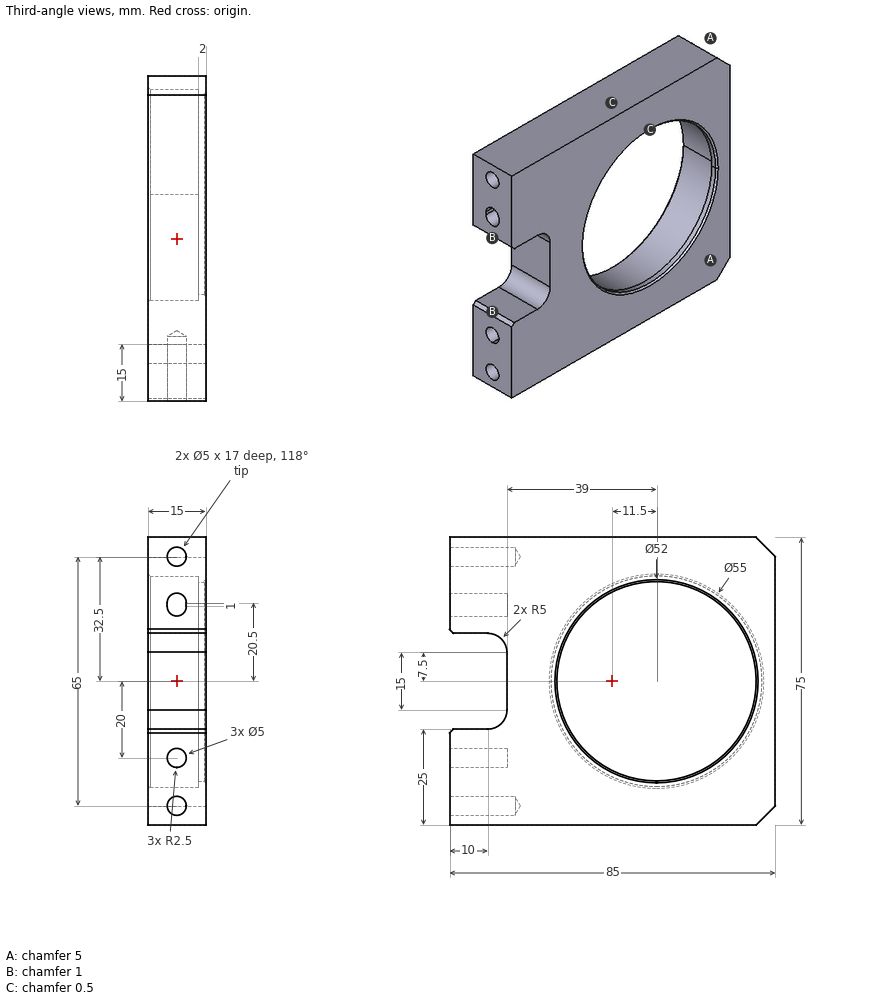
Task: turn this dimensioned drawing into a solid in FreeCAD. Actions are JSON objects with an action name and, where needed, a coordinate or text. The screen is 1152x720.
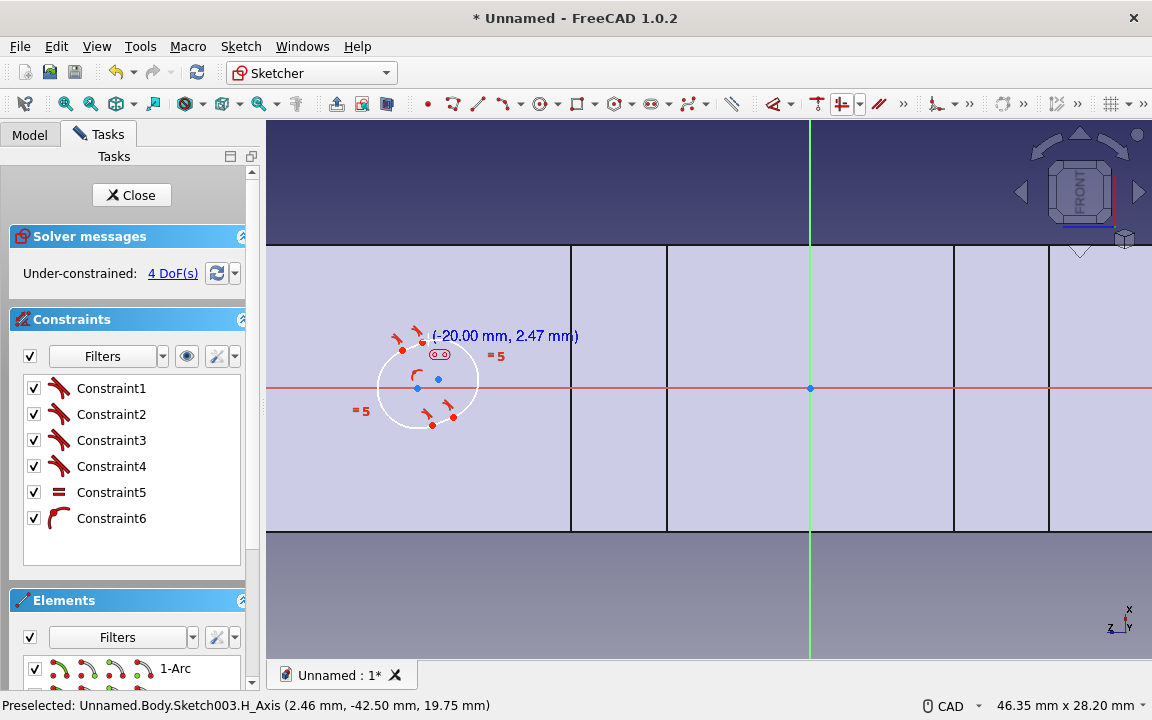
{"action": "left_click", "coordinate": [540, 104]}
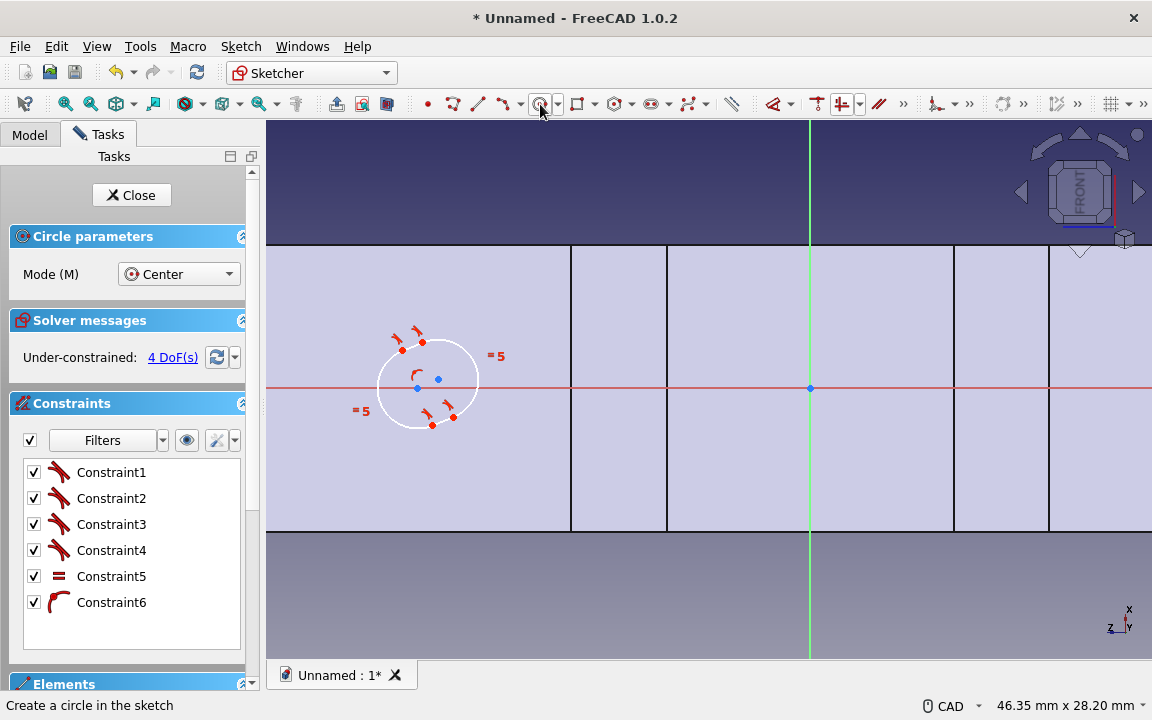
{"action": "scroll", "coordinate": [440, 391], "scroll_direction": "down", "scroll_amount": 3}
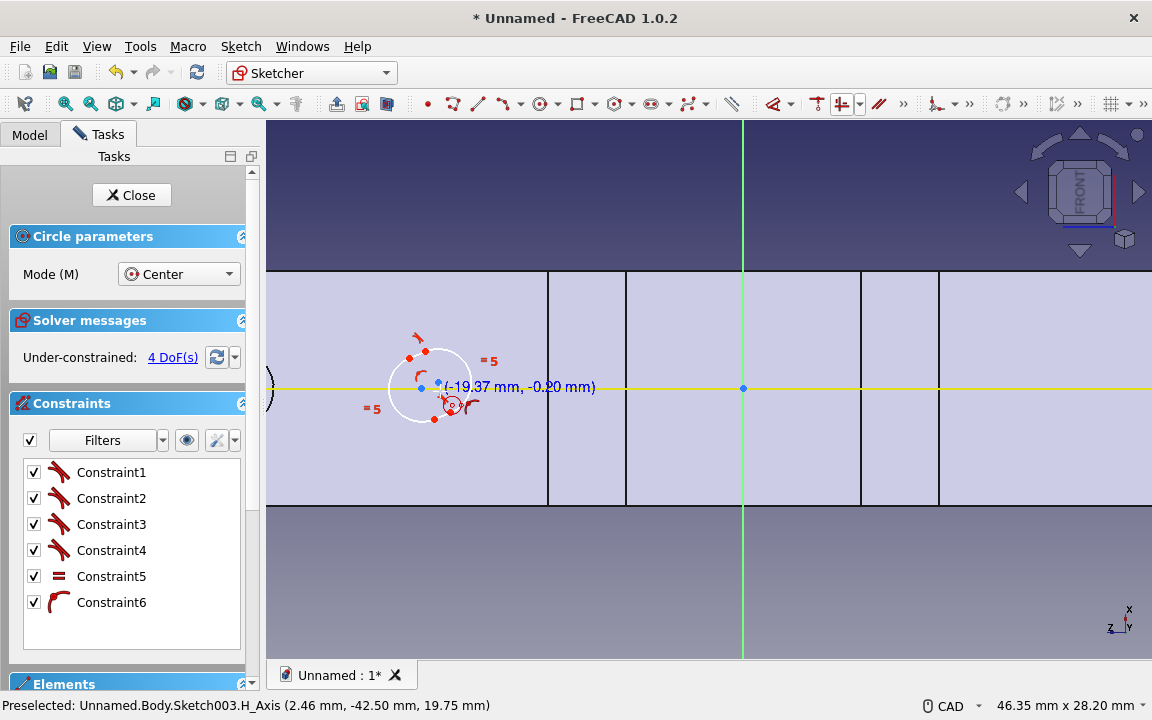
{"action": "left_click", "coordinate": [853, 390]}
{"action": "mouse_move", "coordinate": [872, 371]}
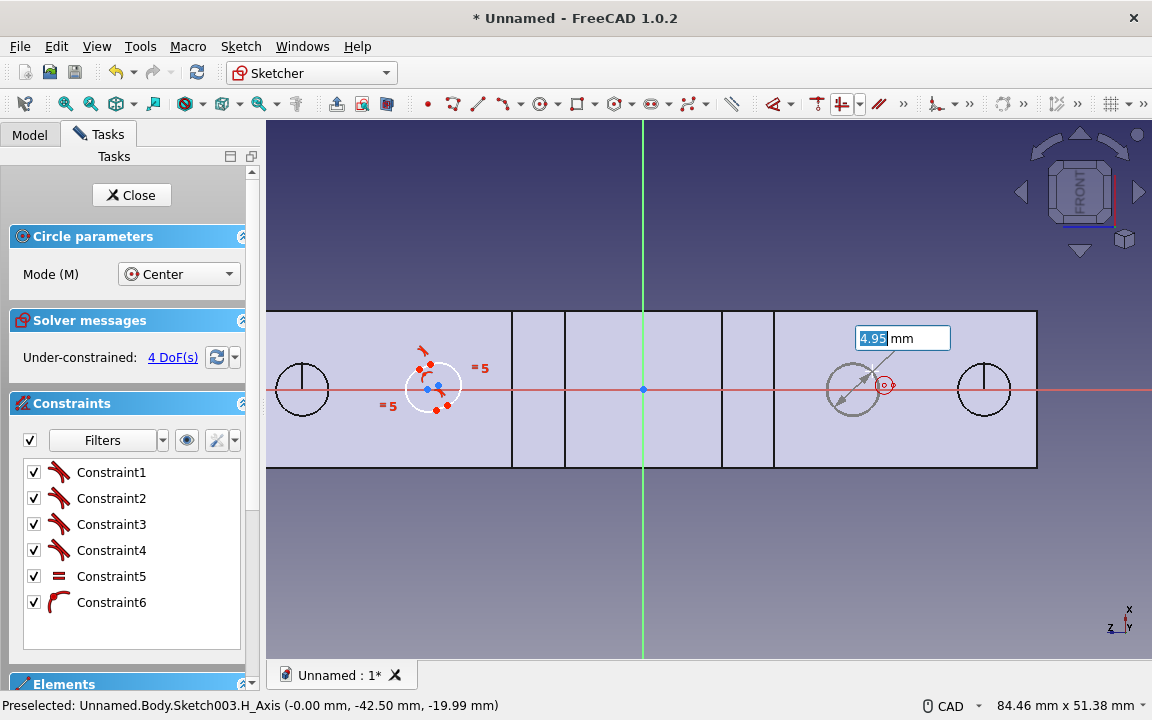
{"action": "type", "text": "5"}
{"action": "key", "text": "Return"}
{"action": "key", "text": "Escape"}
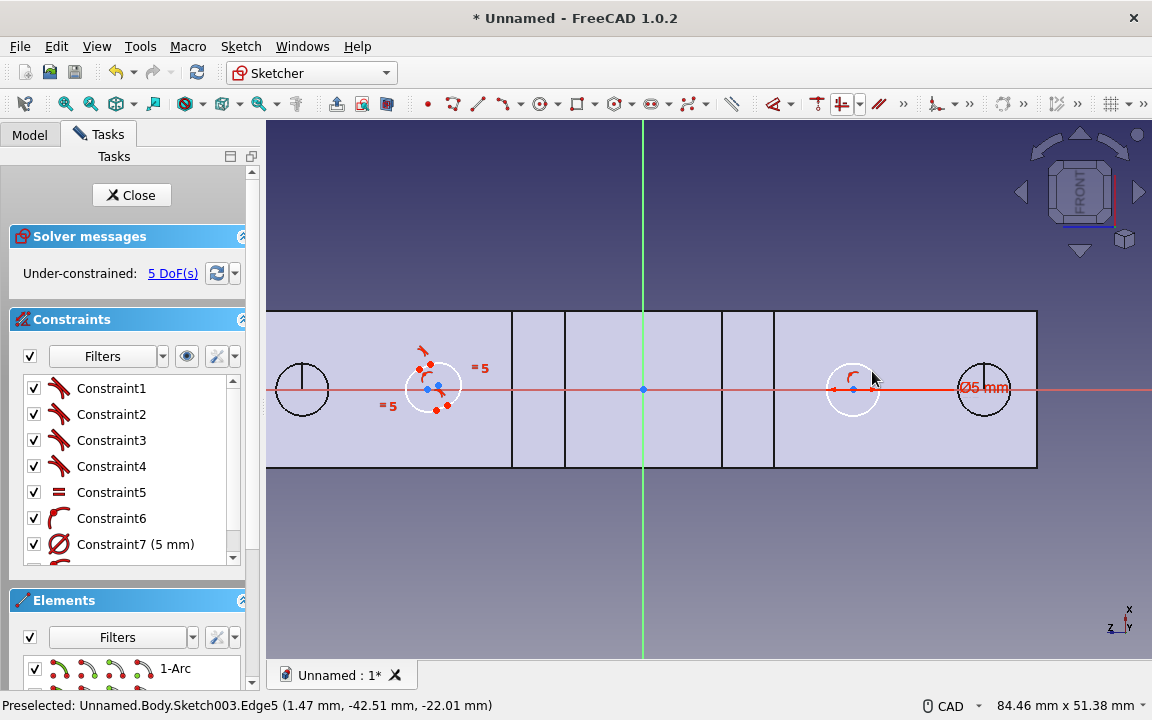
{"action": "left_click", "coordinate": [439, 385]}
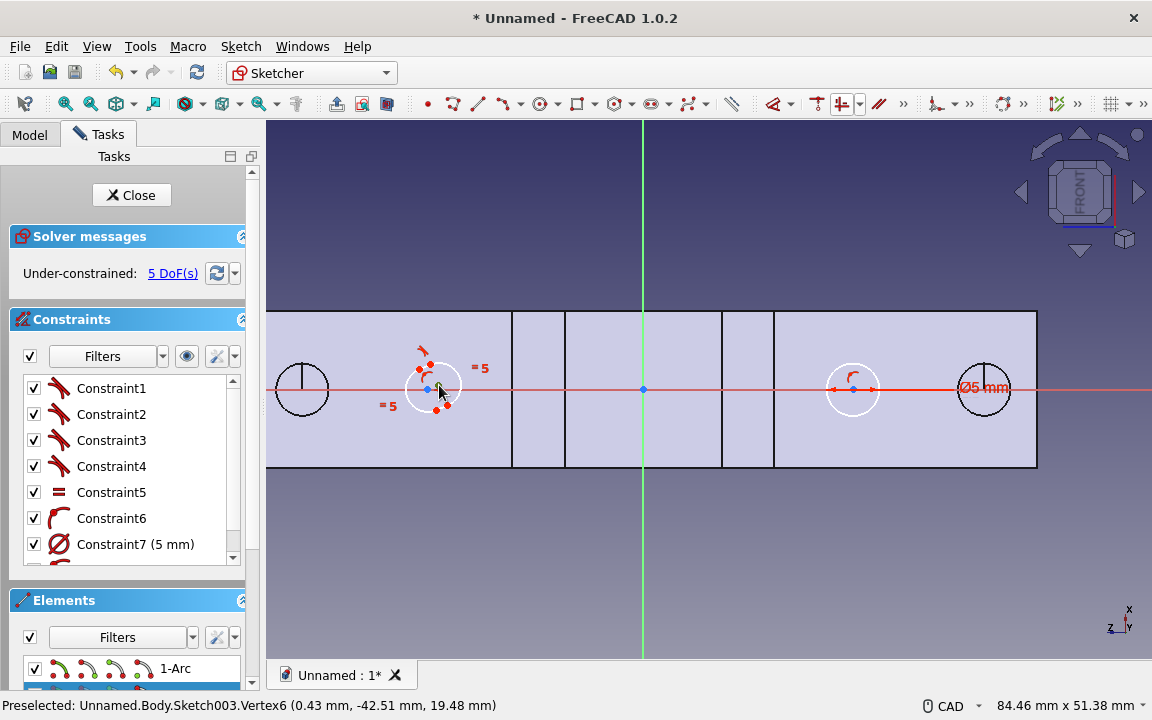
{"action": "left_click", "coordinate": [344, 390]}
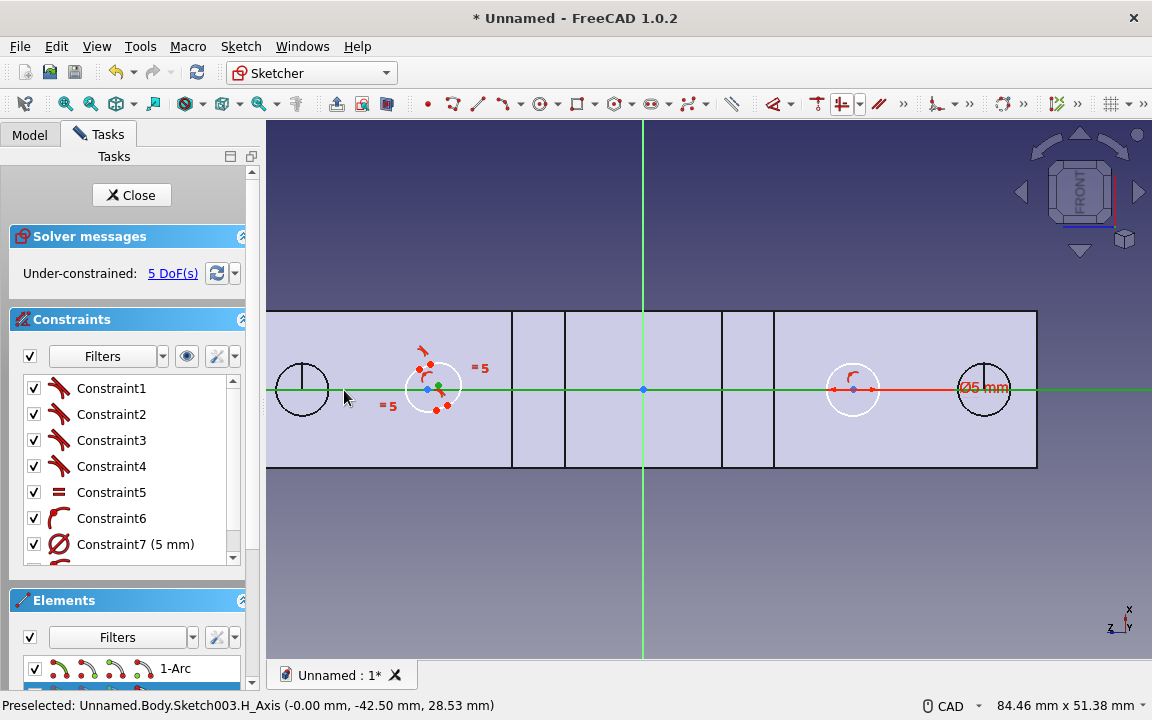
{"action": "left_click", "coordinate": [817, 104]}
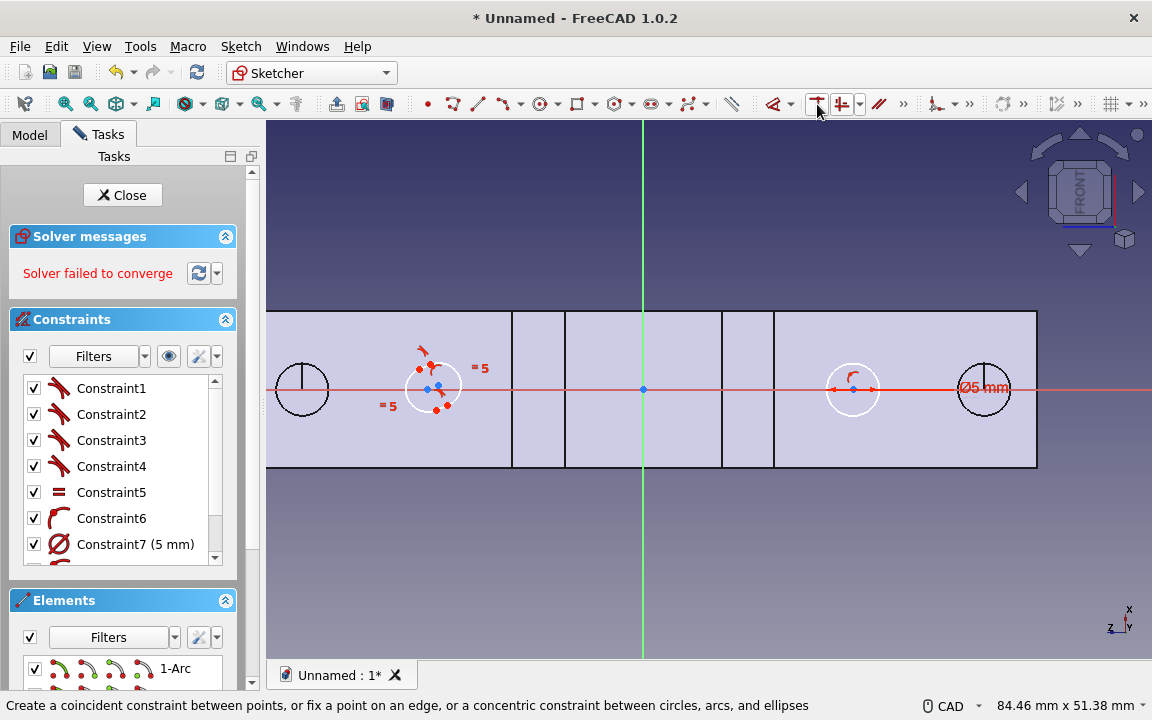
{"action": "left_click", "coordinate": [772, 104]}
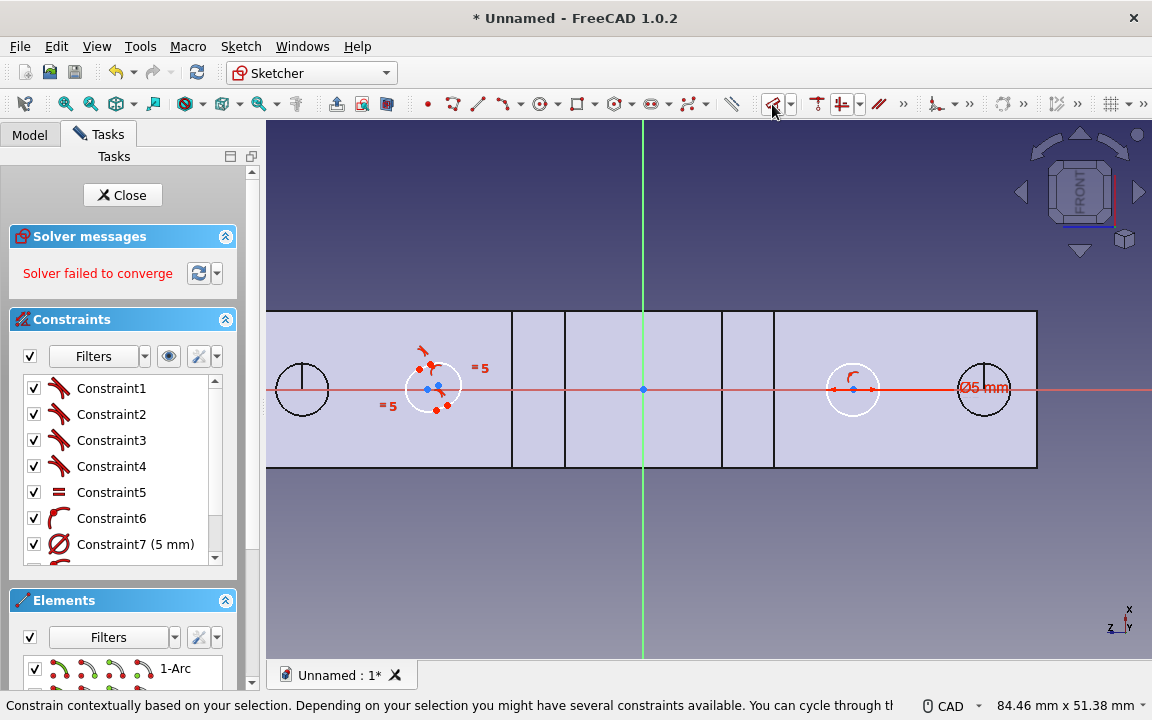
{"action": "scroll", "coordinate": [416, 408], "scroll_direction": "up", "scroll_amount": 3}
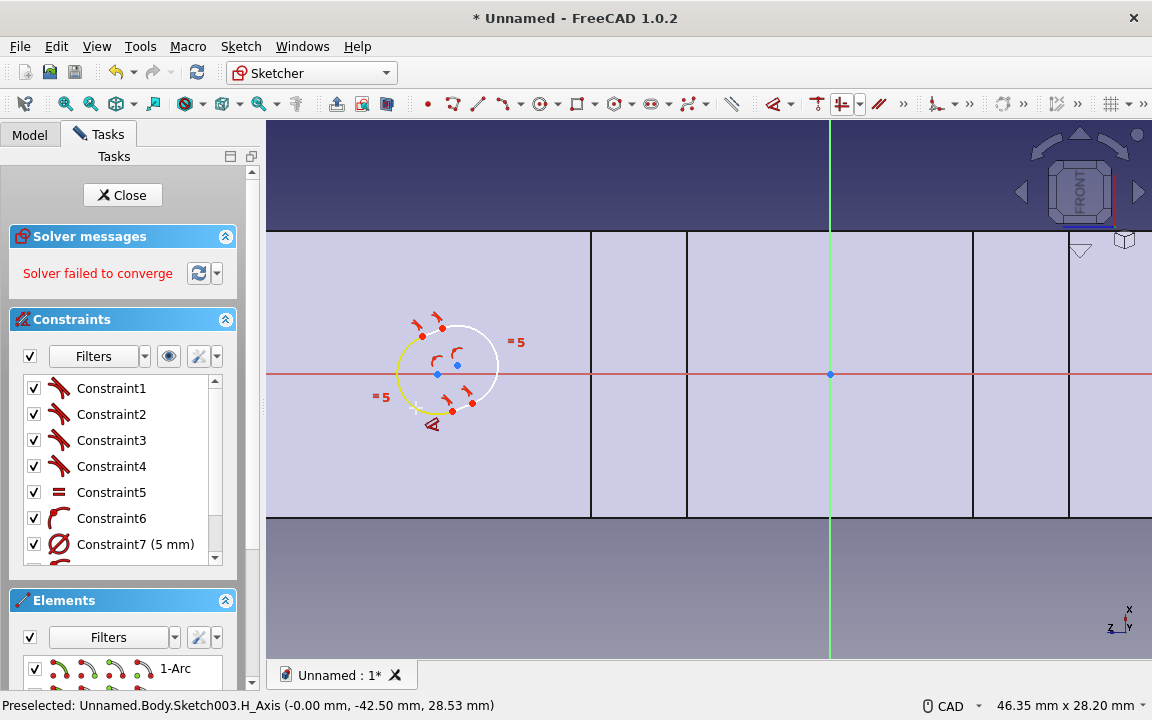
{"action": "left_click", "coordinate": [416, 408]}
{"action": "left_click", "coordinate": [399, 435]}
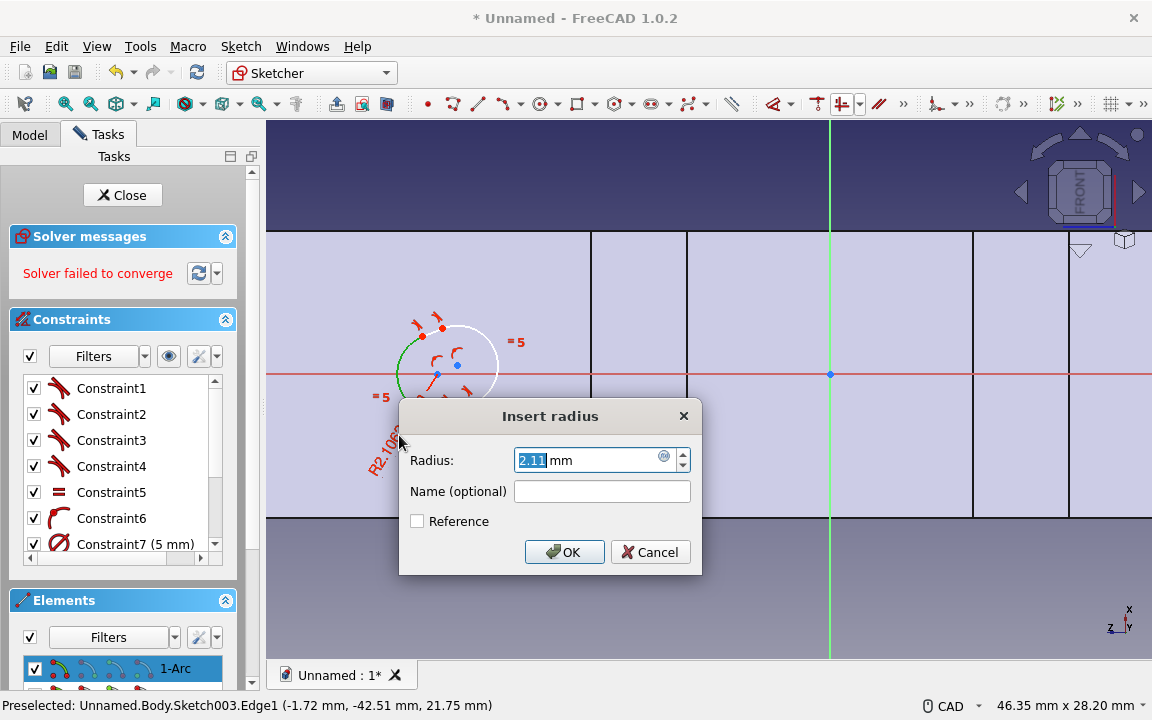
{"action": "type", "text": "2.5"}
{"action": "key", "text": "Return"}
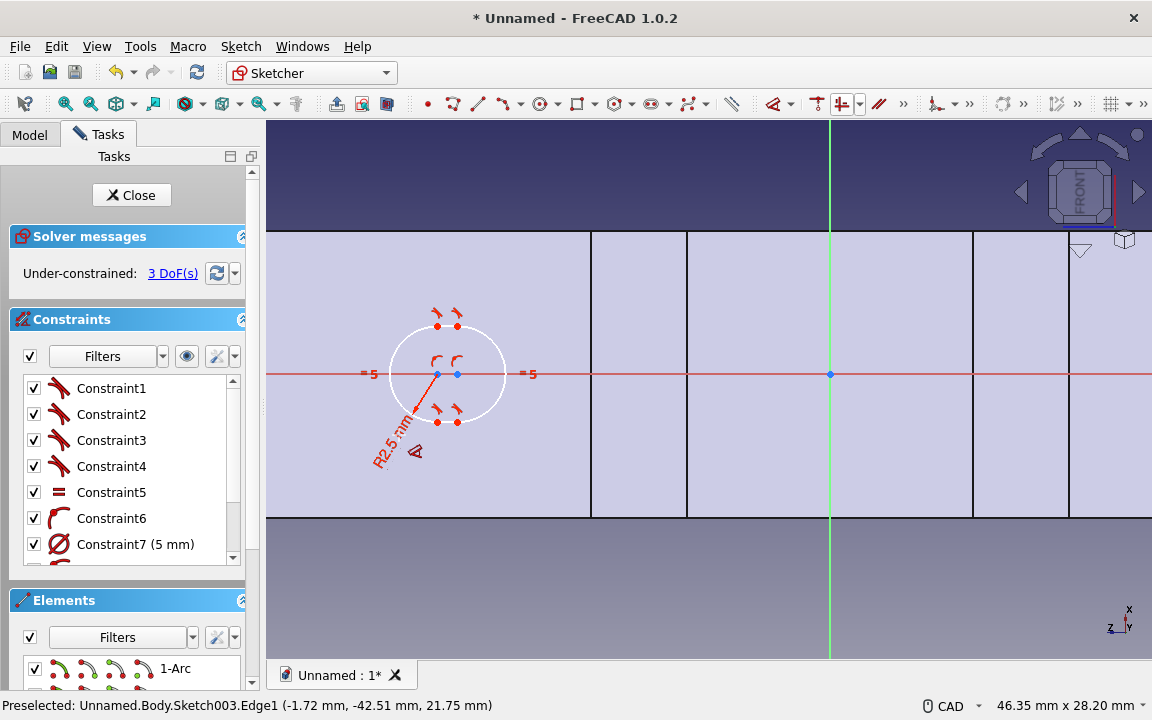
{"action": "scroll", "coordinate": [448, 326], "scroll_direction": "up", "scroll_amount": 4}